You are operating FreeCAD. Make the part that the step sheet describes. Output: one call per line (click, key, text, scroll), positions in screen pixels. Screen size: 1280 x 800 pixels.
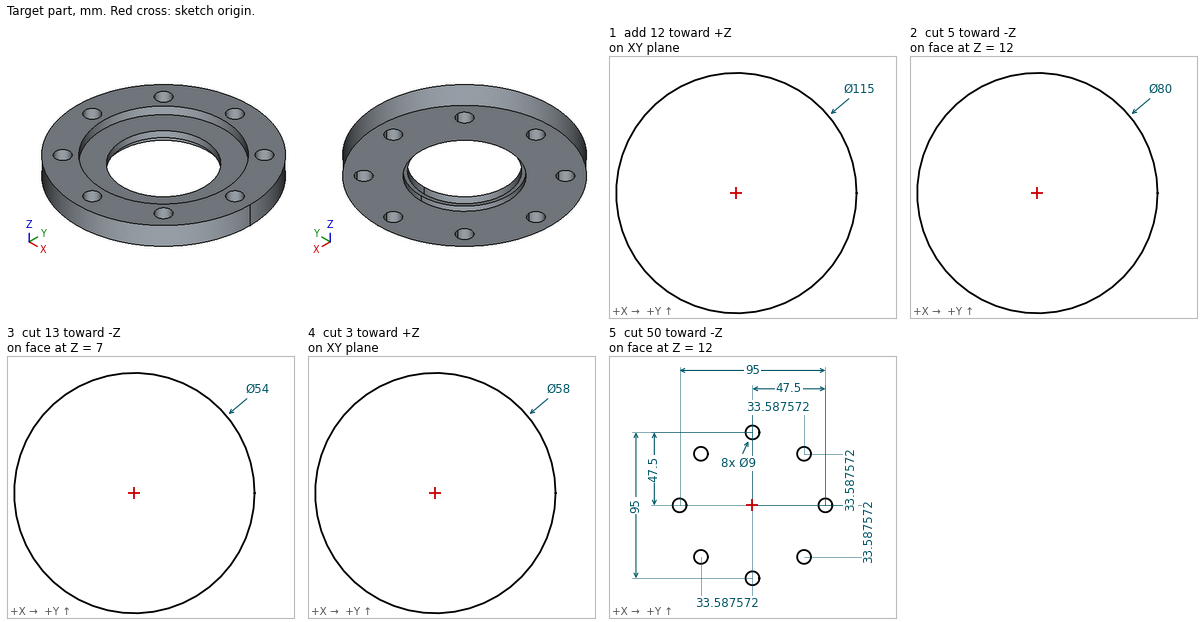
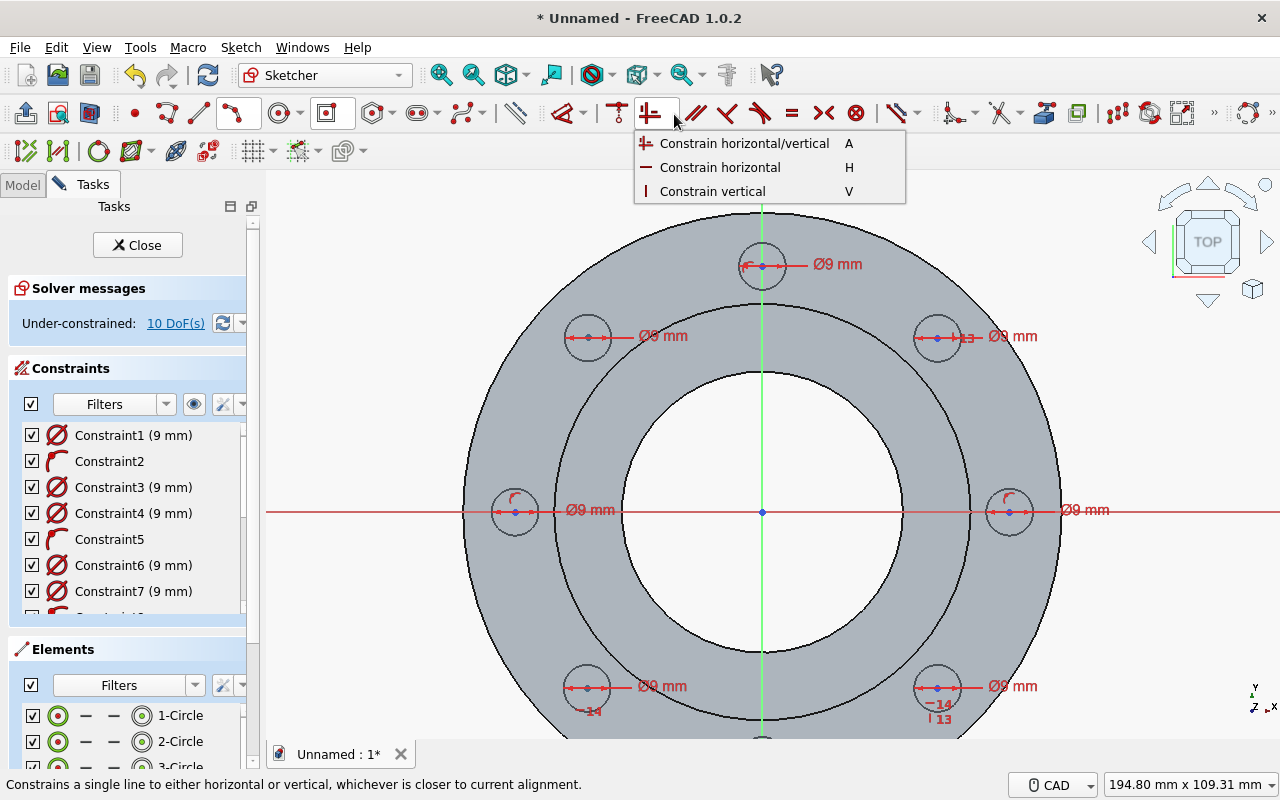
click(770, 191)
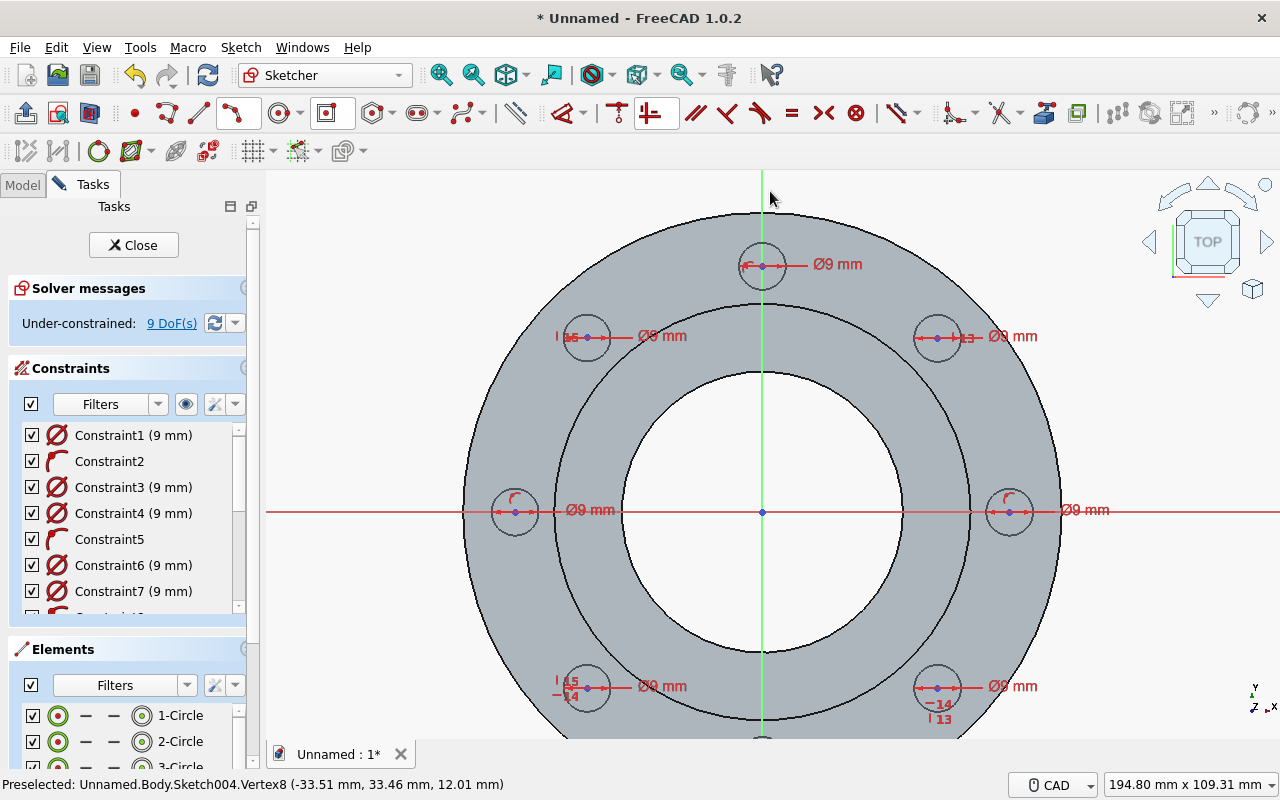
click(938, 338)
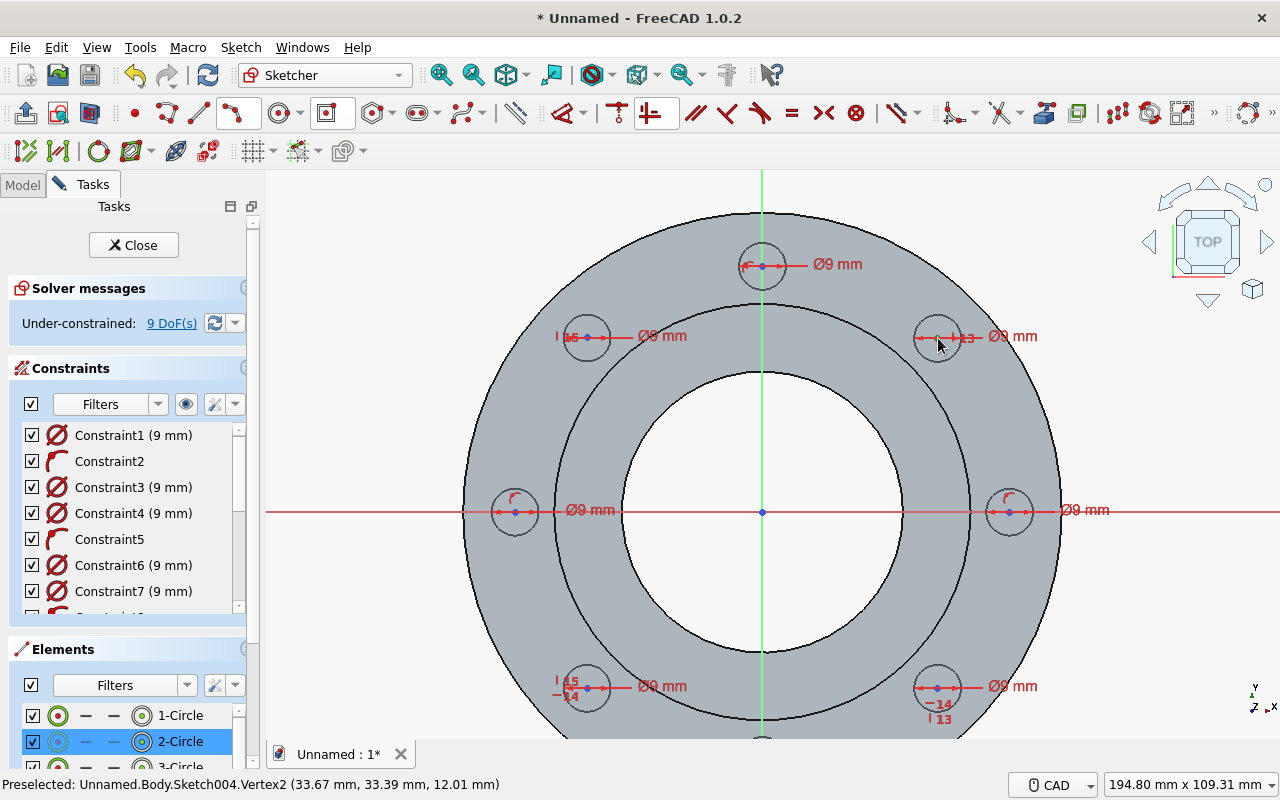
click(587, 338)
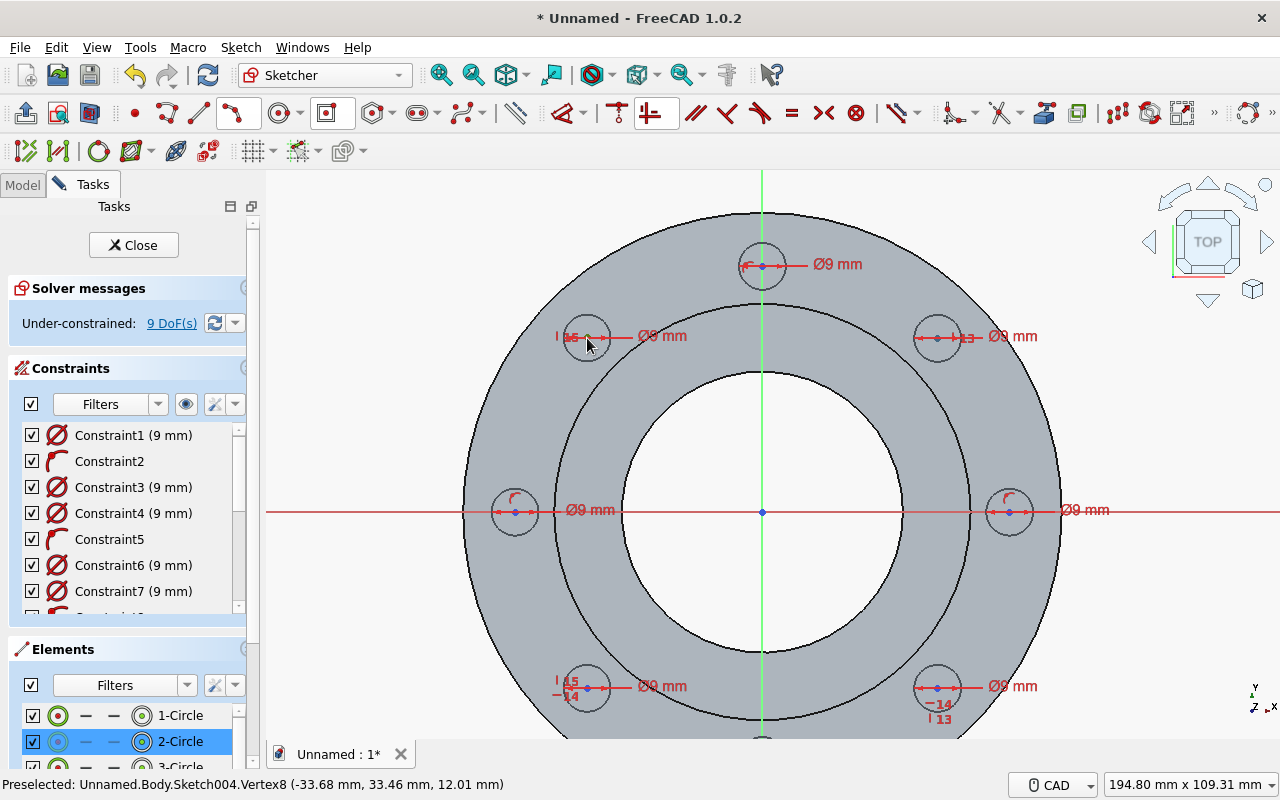
click(674, 114)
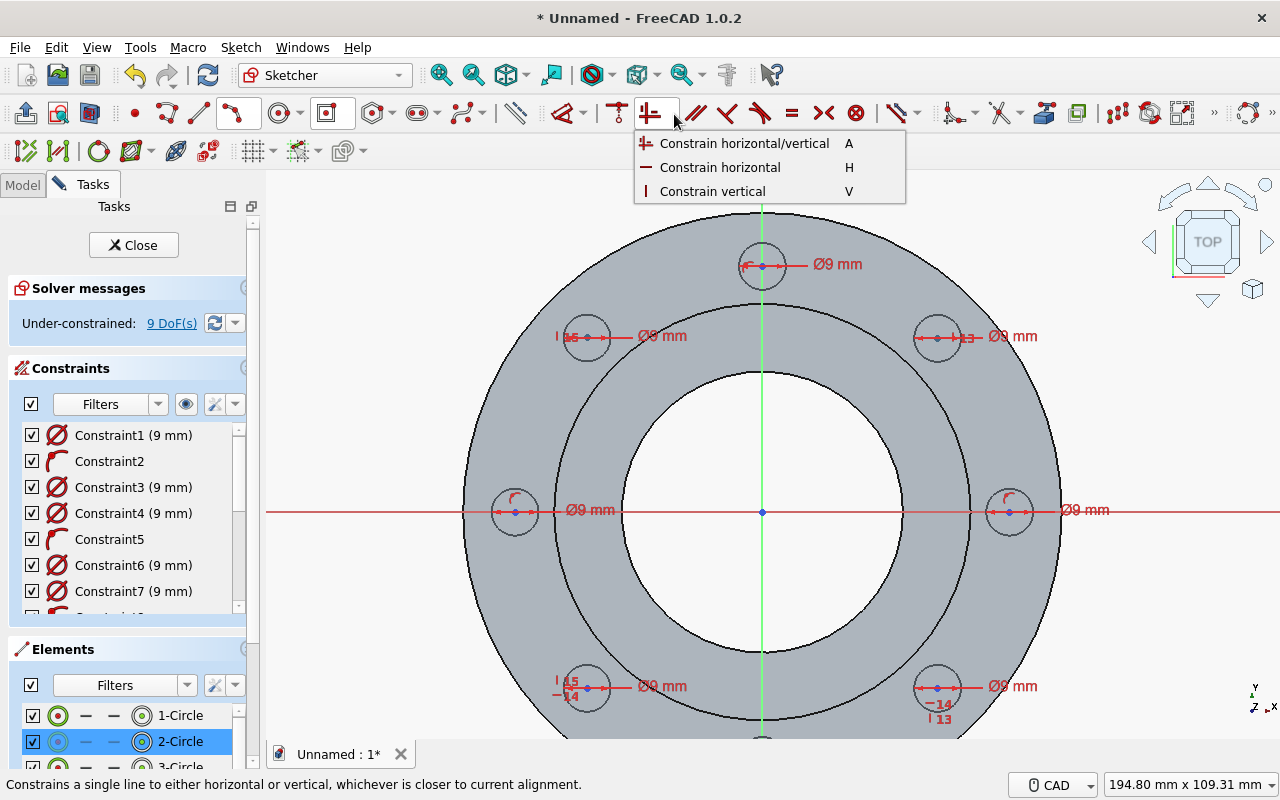
click(770, 167)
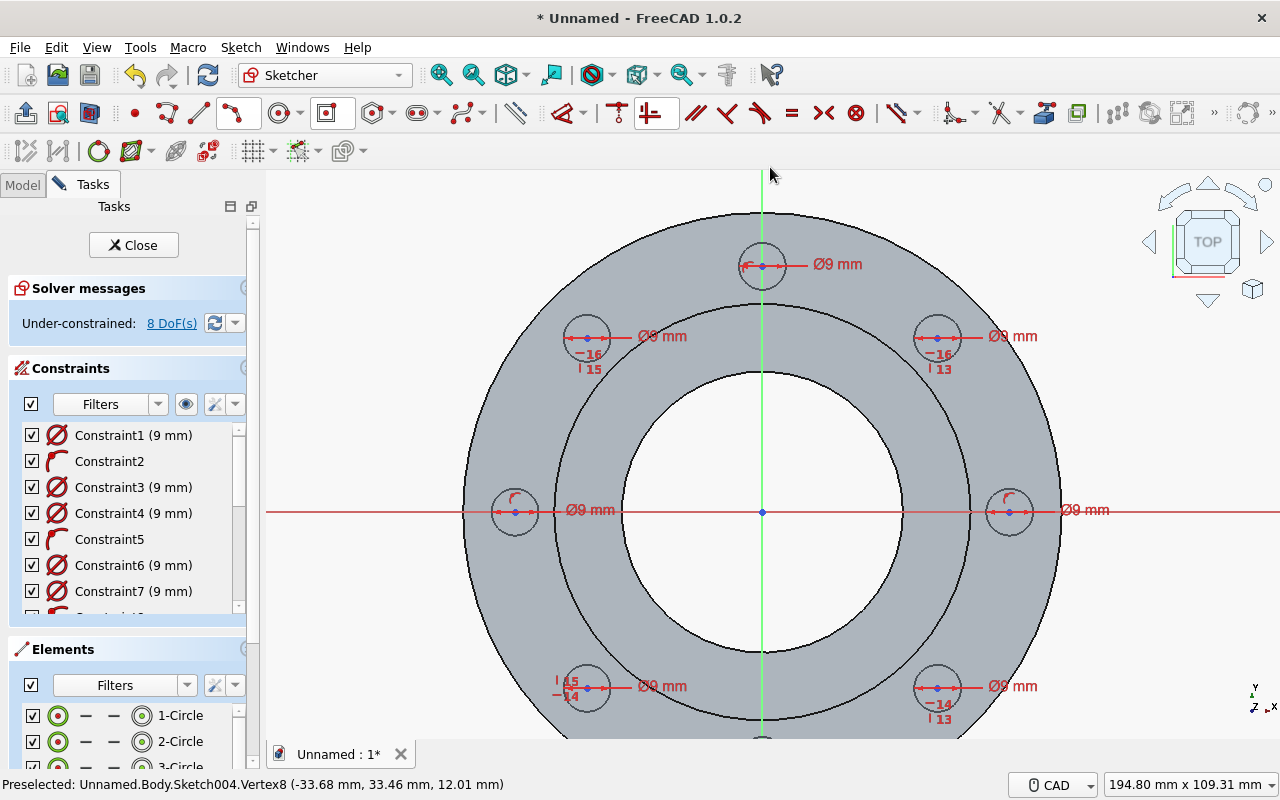
click(562, 114)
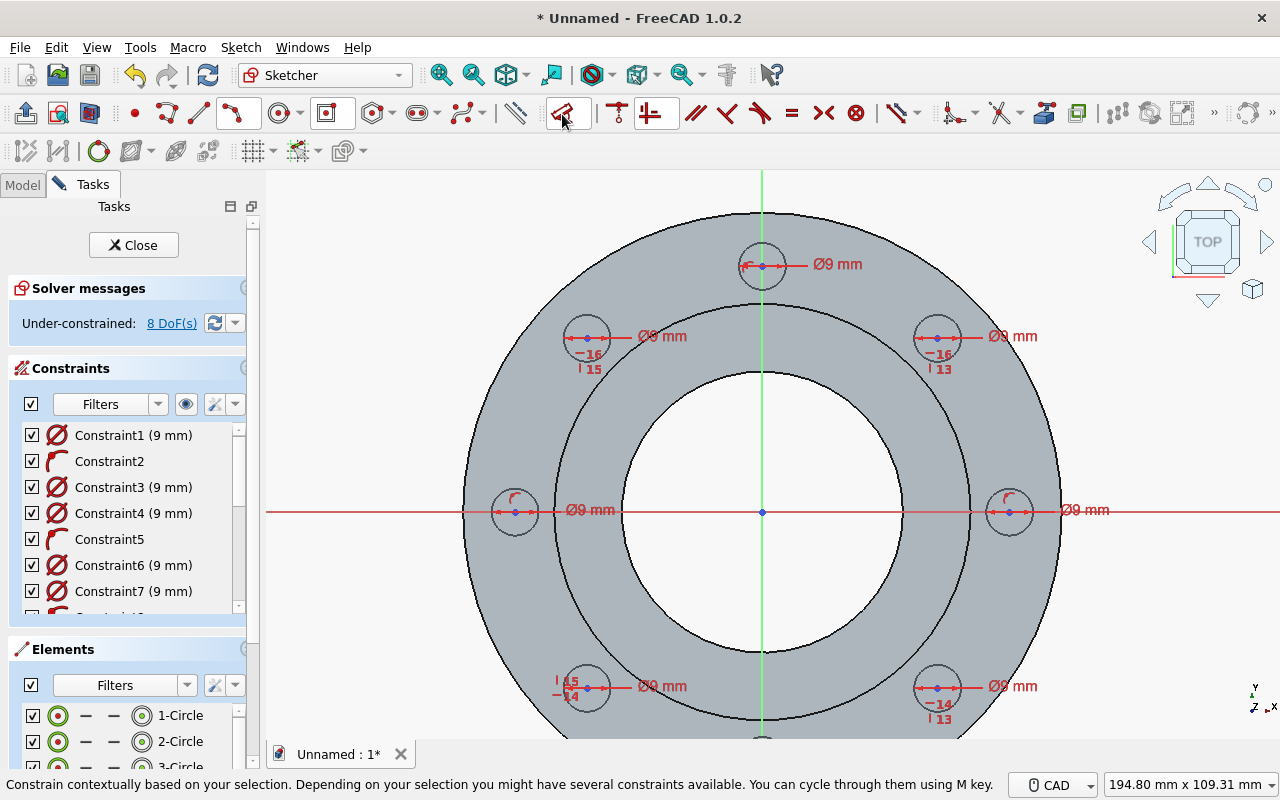
click(762, 266)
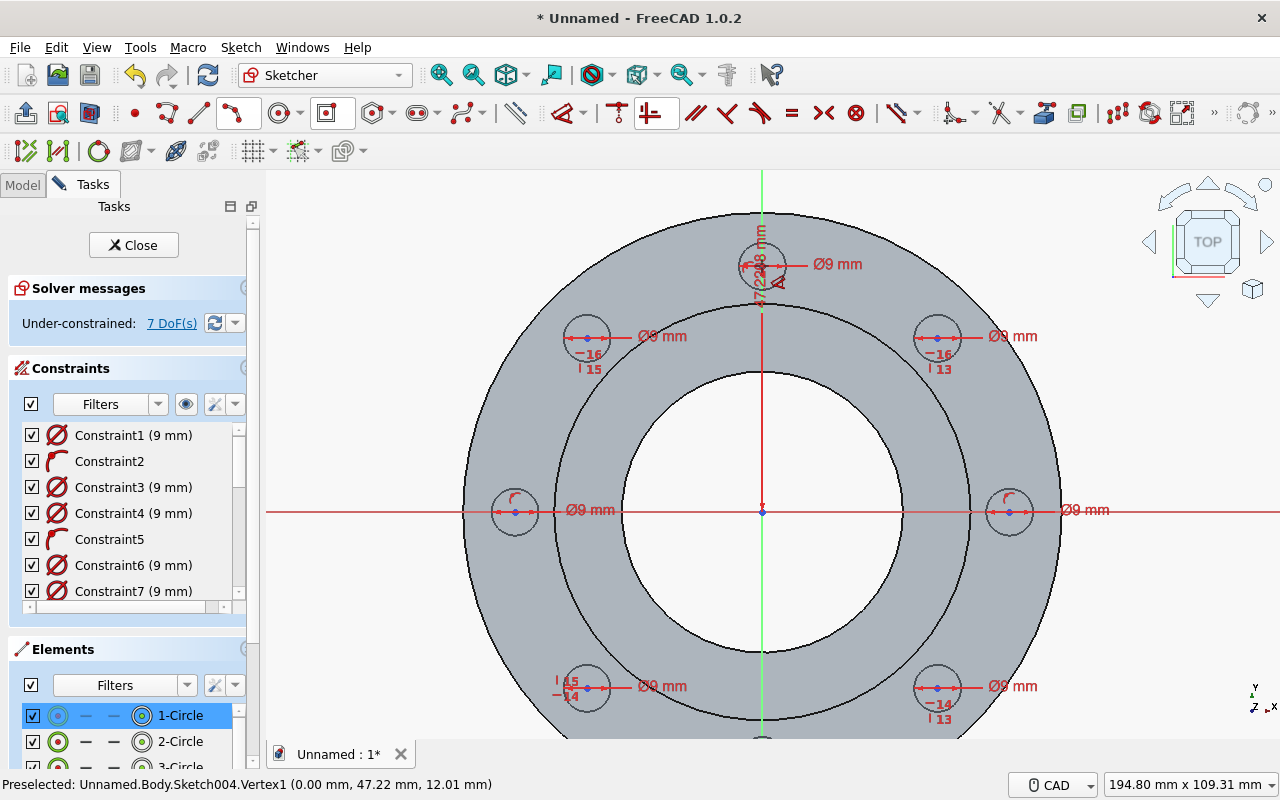
scroll(587, 337, down, 2)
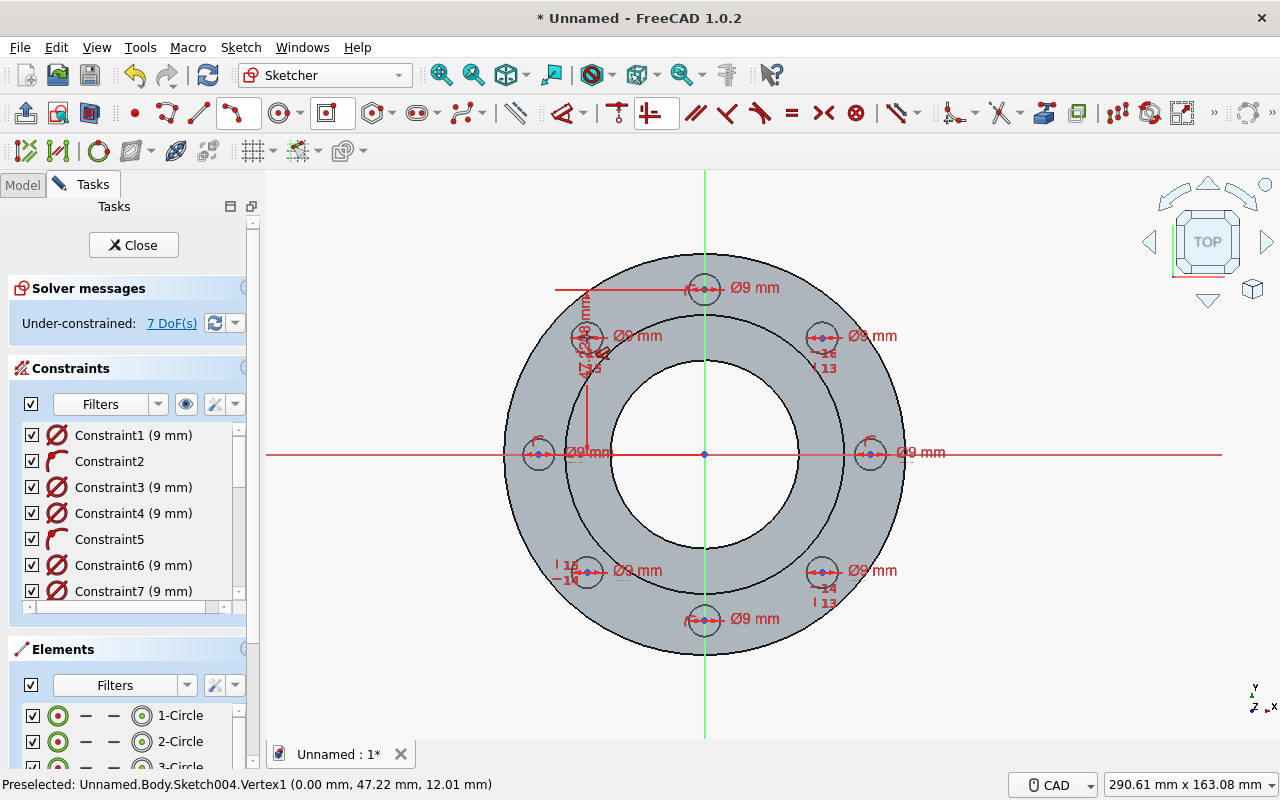
click(705, 621)
click(739, 379)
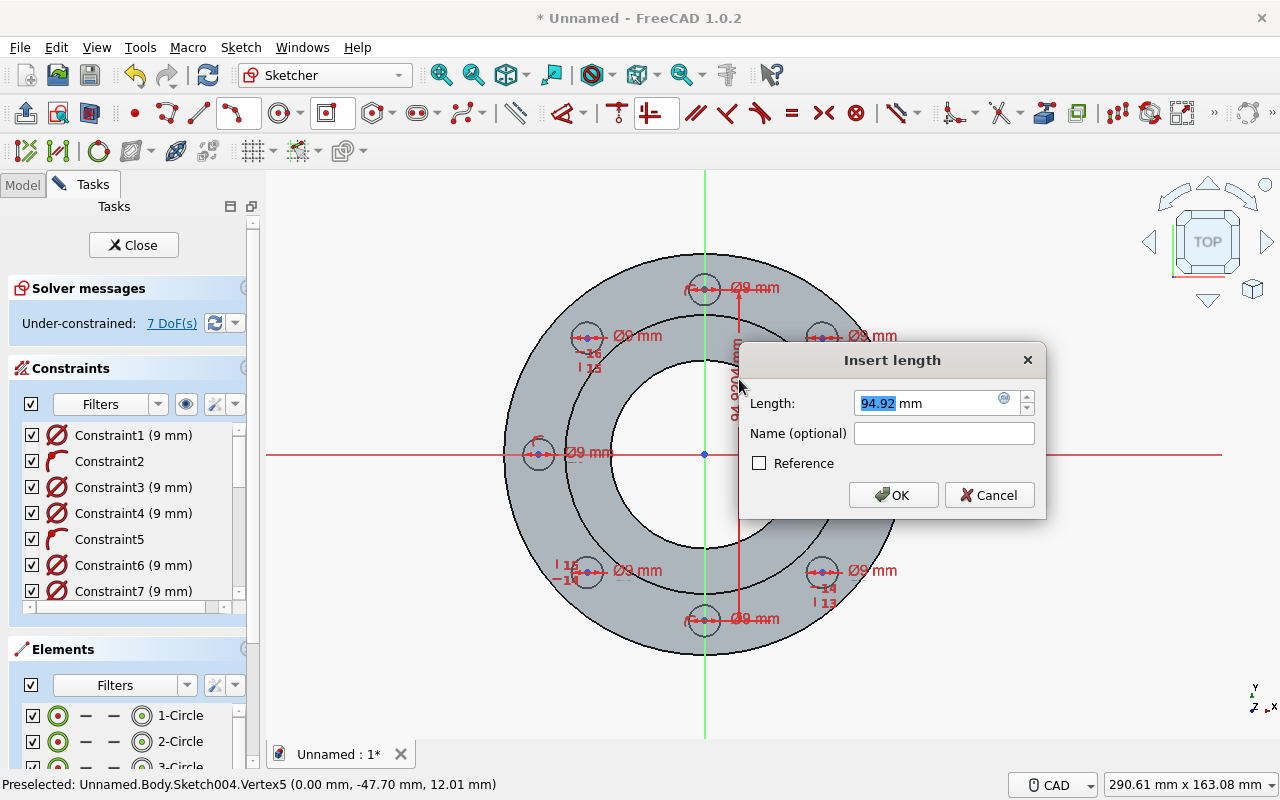
text(95)
key(Return)